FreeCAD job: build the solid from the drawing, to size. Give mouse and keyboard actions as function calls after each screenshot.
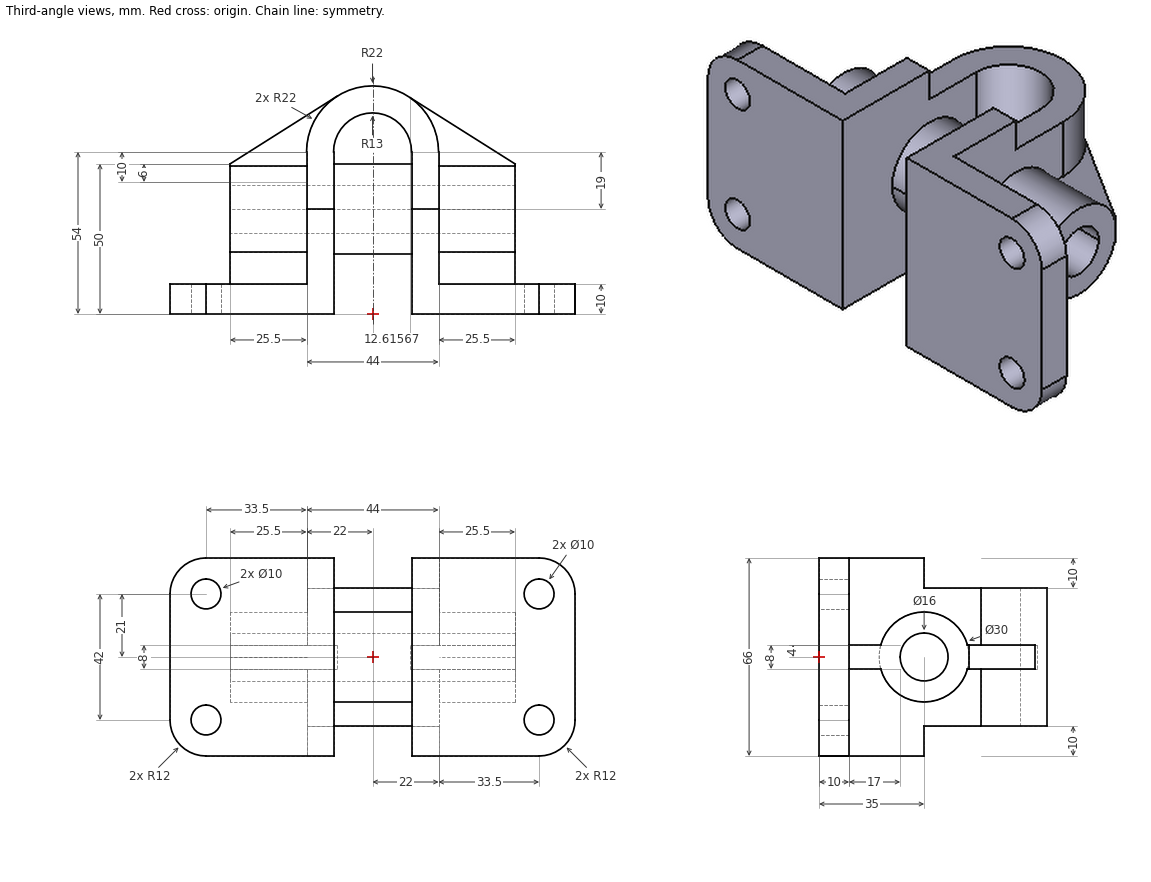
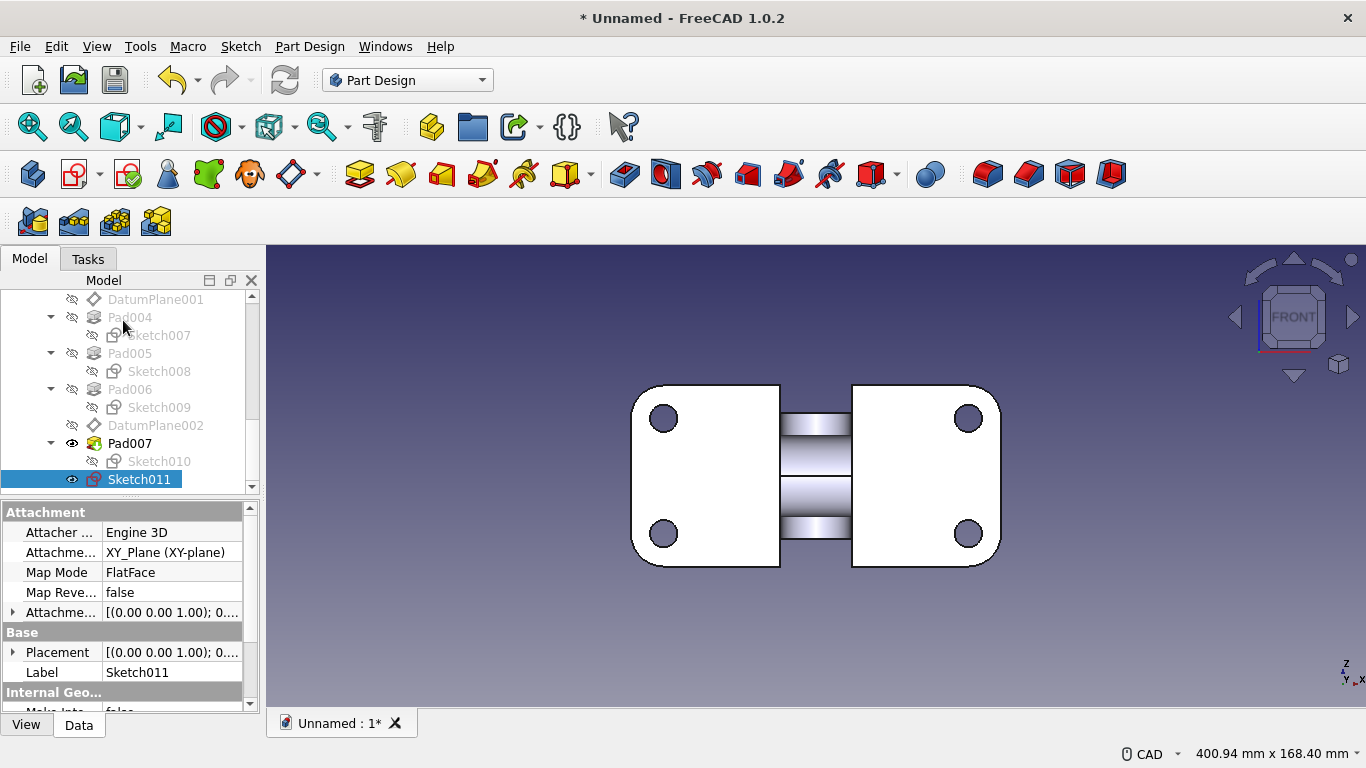
click(360, 174)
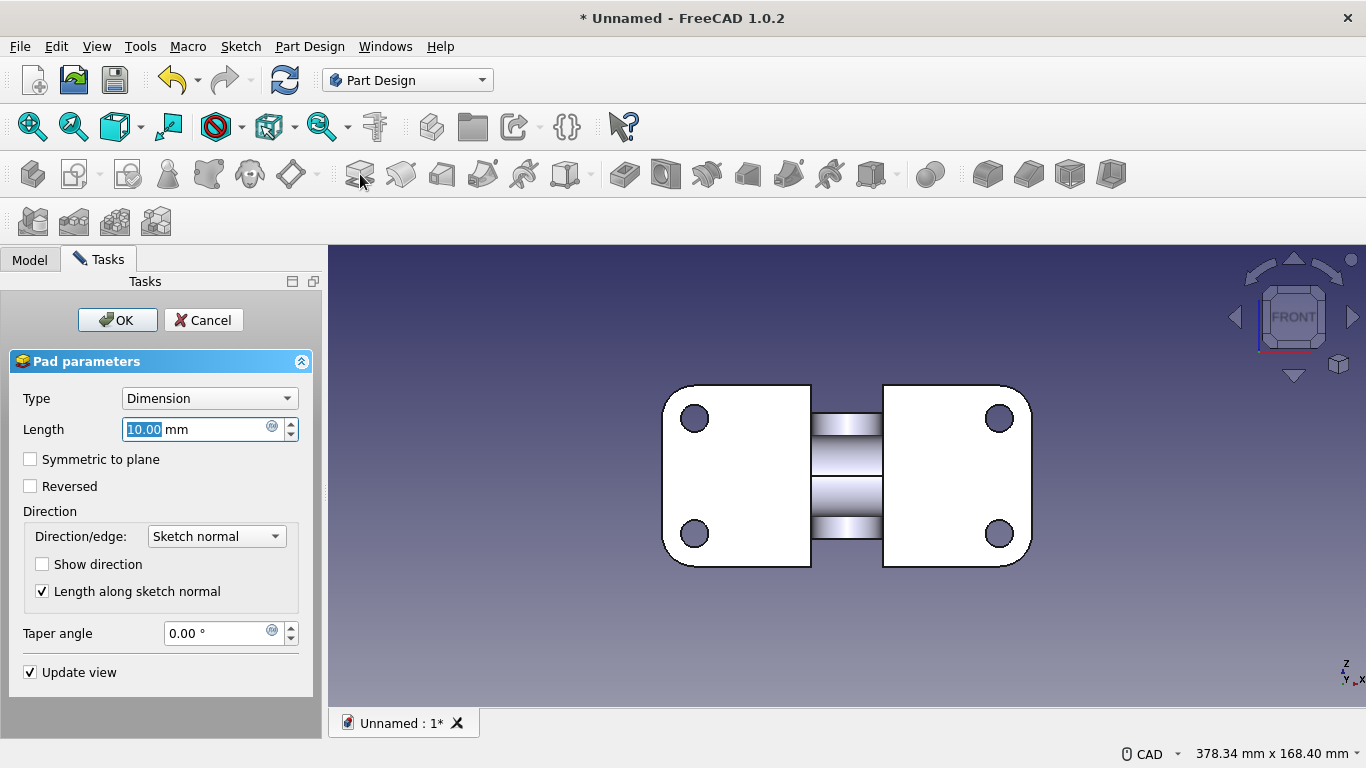
text(8)
key(Tab)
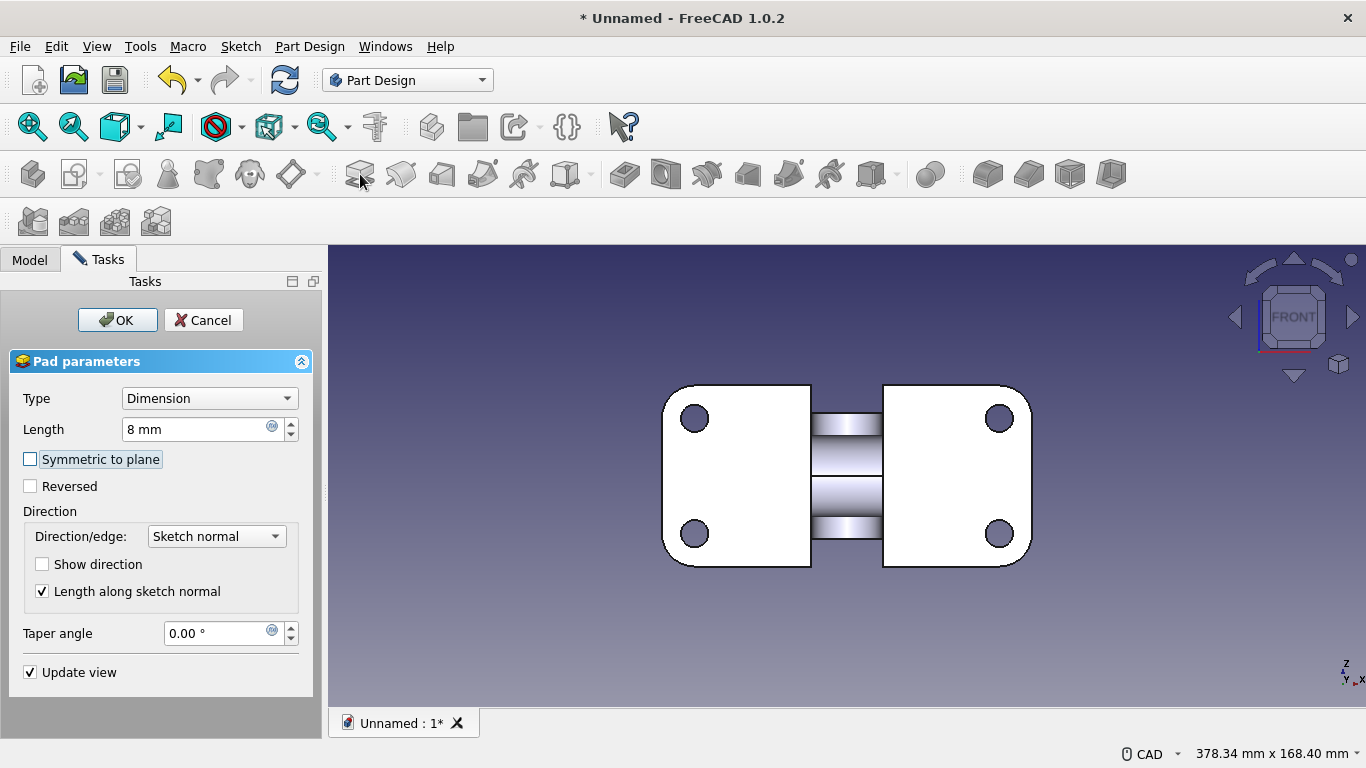
click(31, 459)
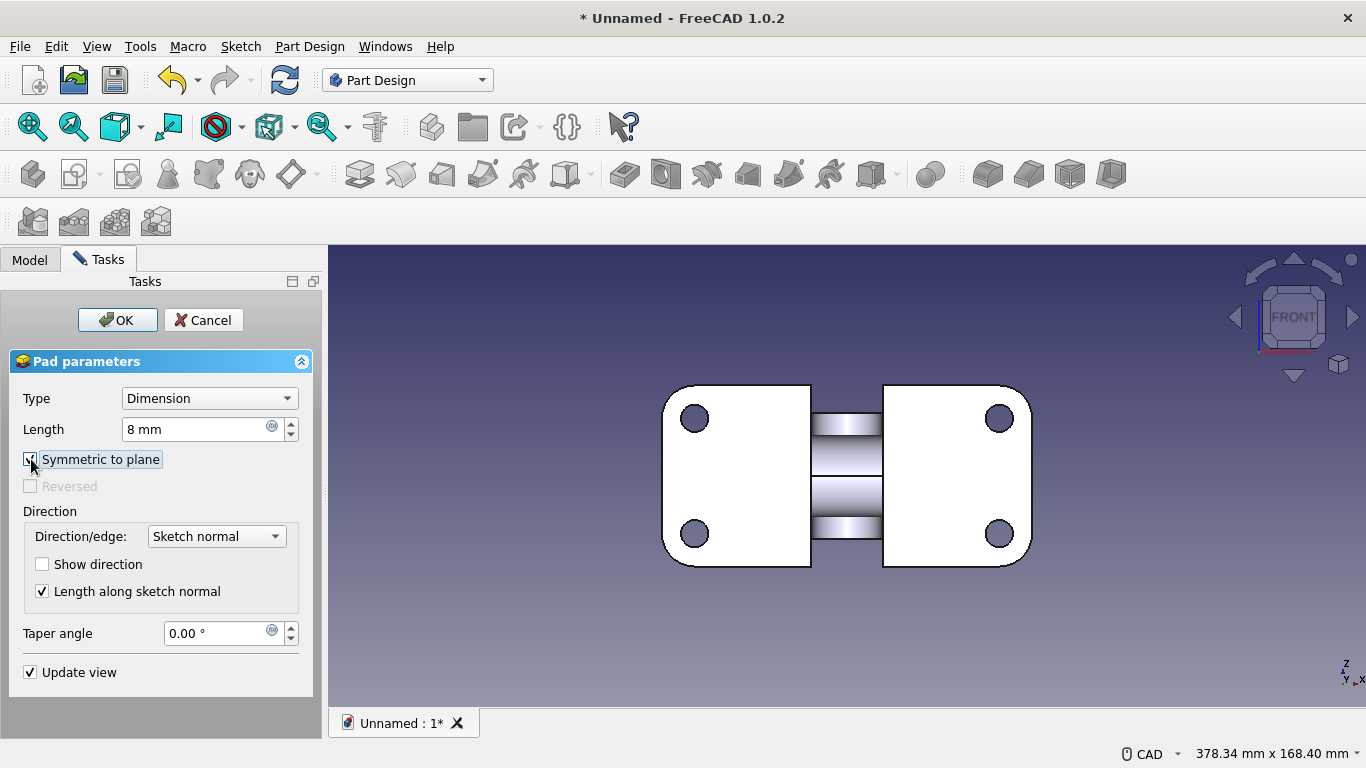
click(118, 320)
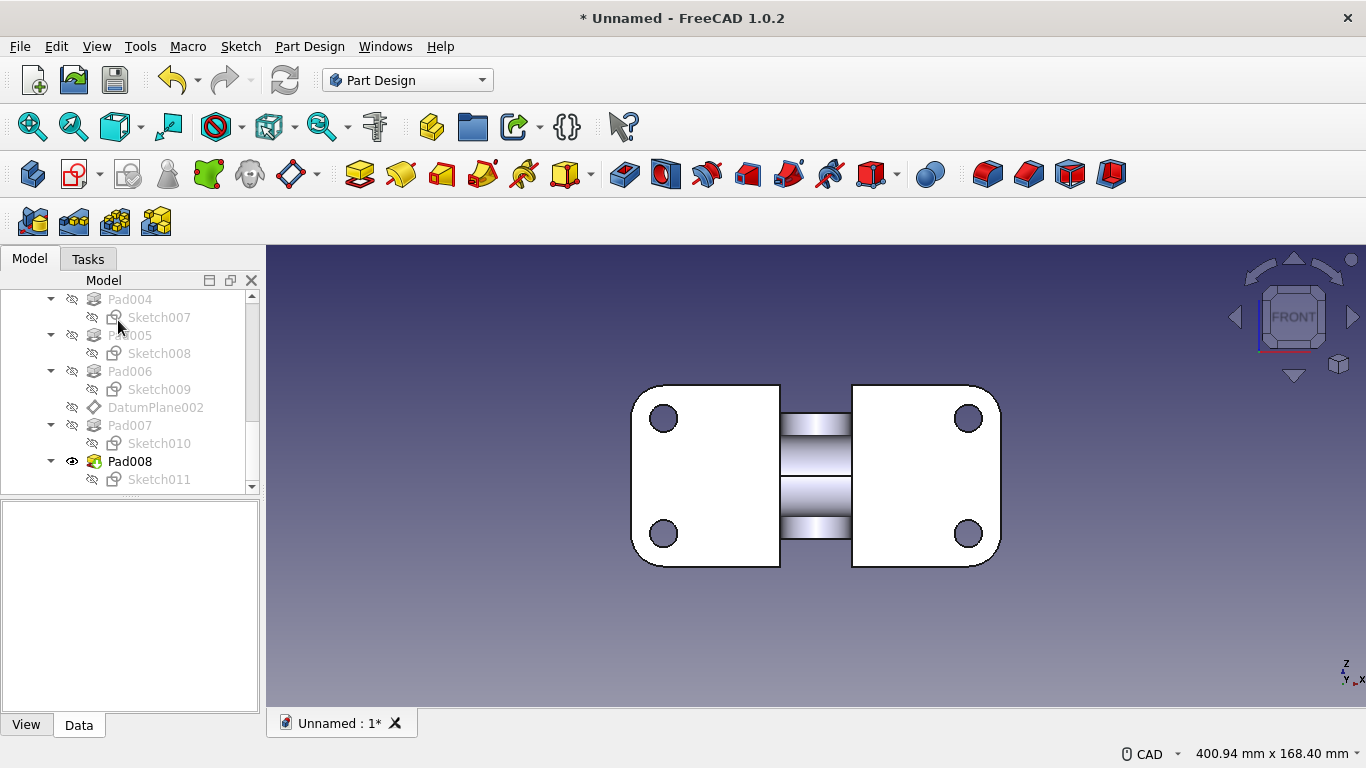
key(0)